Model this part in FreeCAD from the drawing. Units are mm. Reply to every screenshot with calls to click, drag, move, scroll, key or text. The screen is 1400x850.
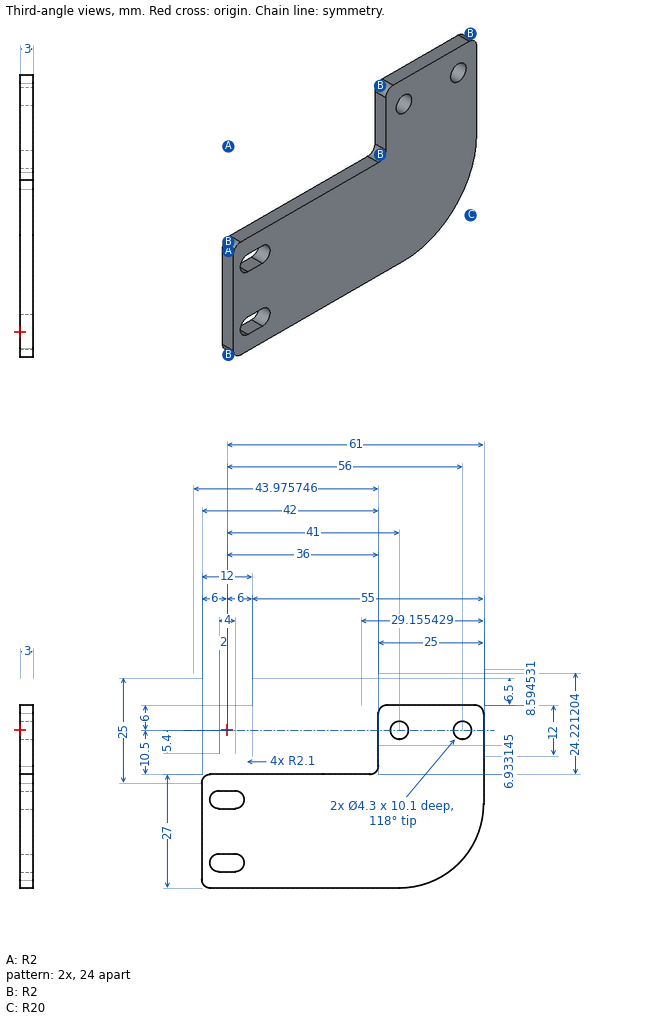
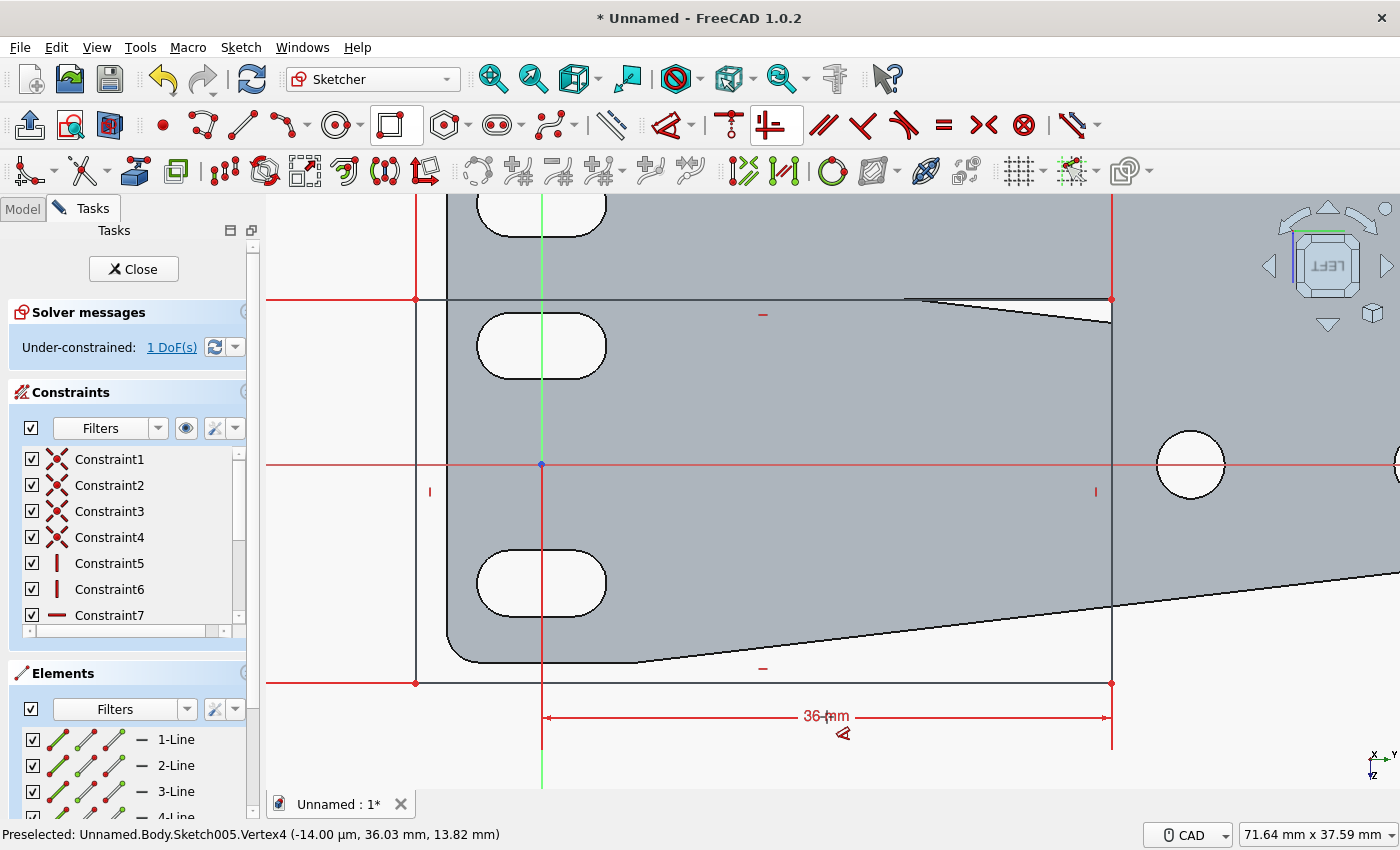
click(416, 300)
click(382, 382)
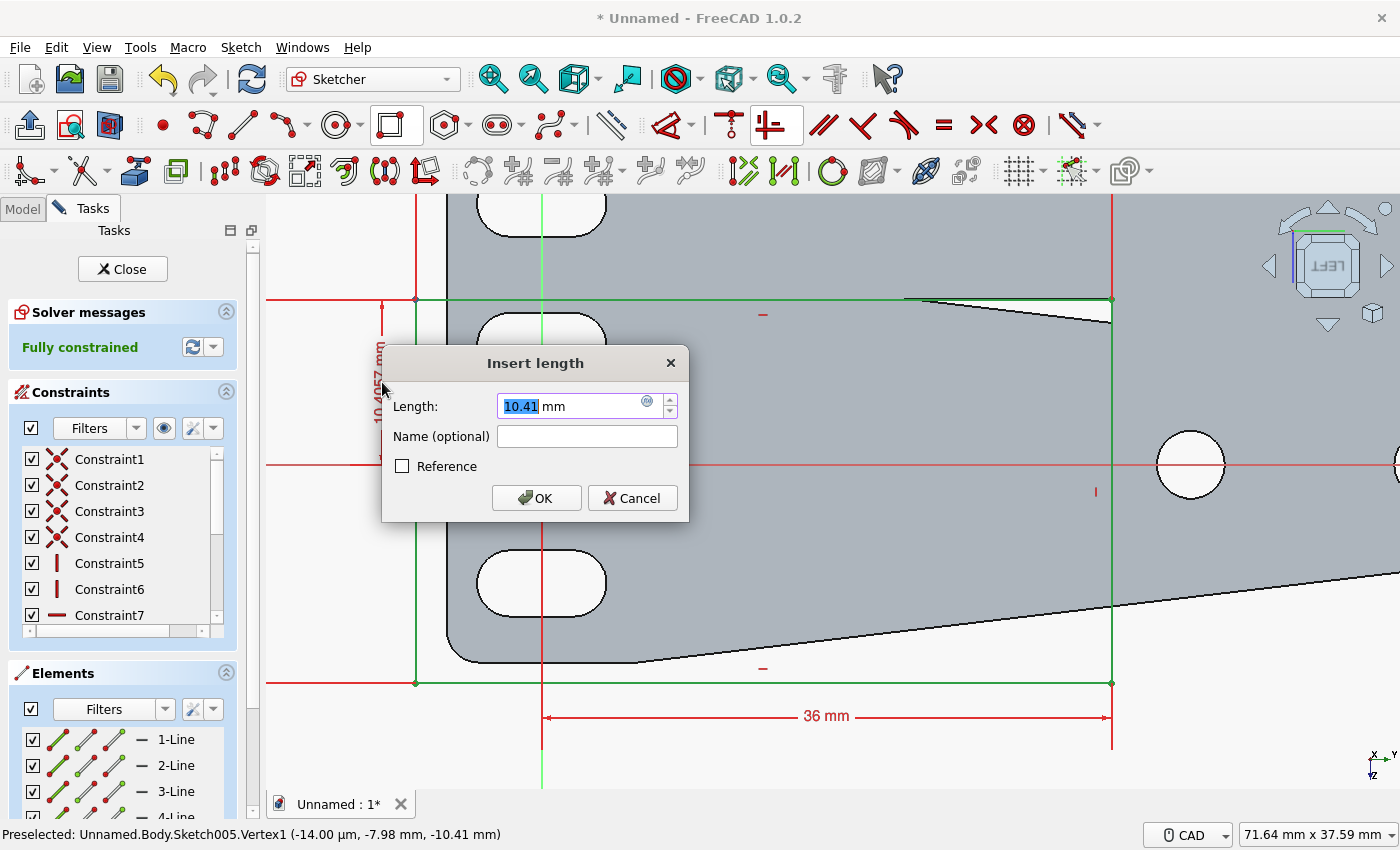
text(10.5)
key(Return)
key(Escape)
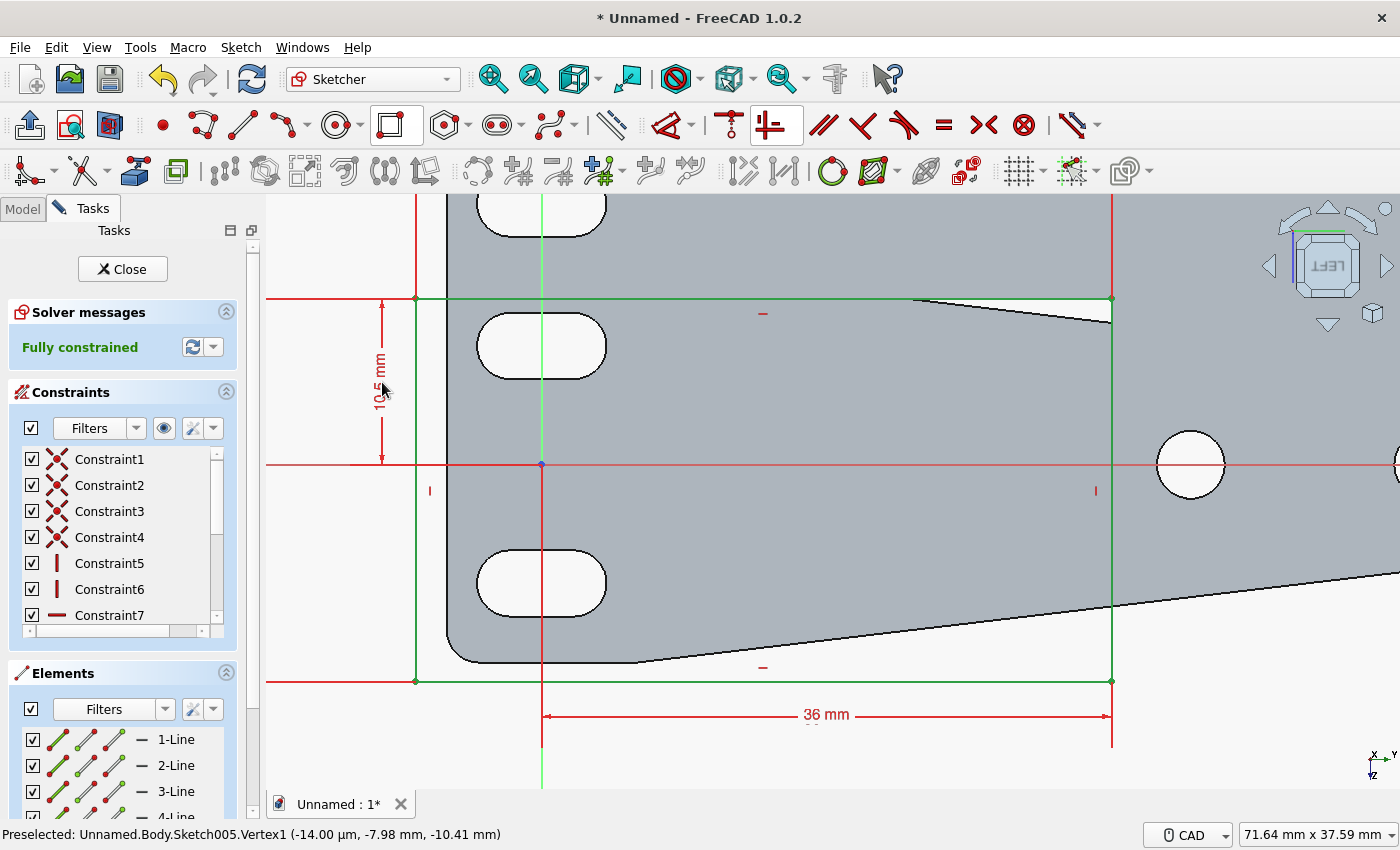
click(123, 269)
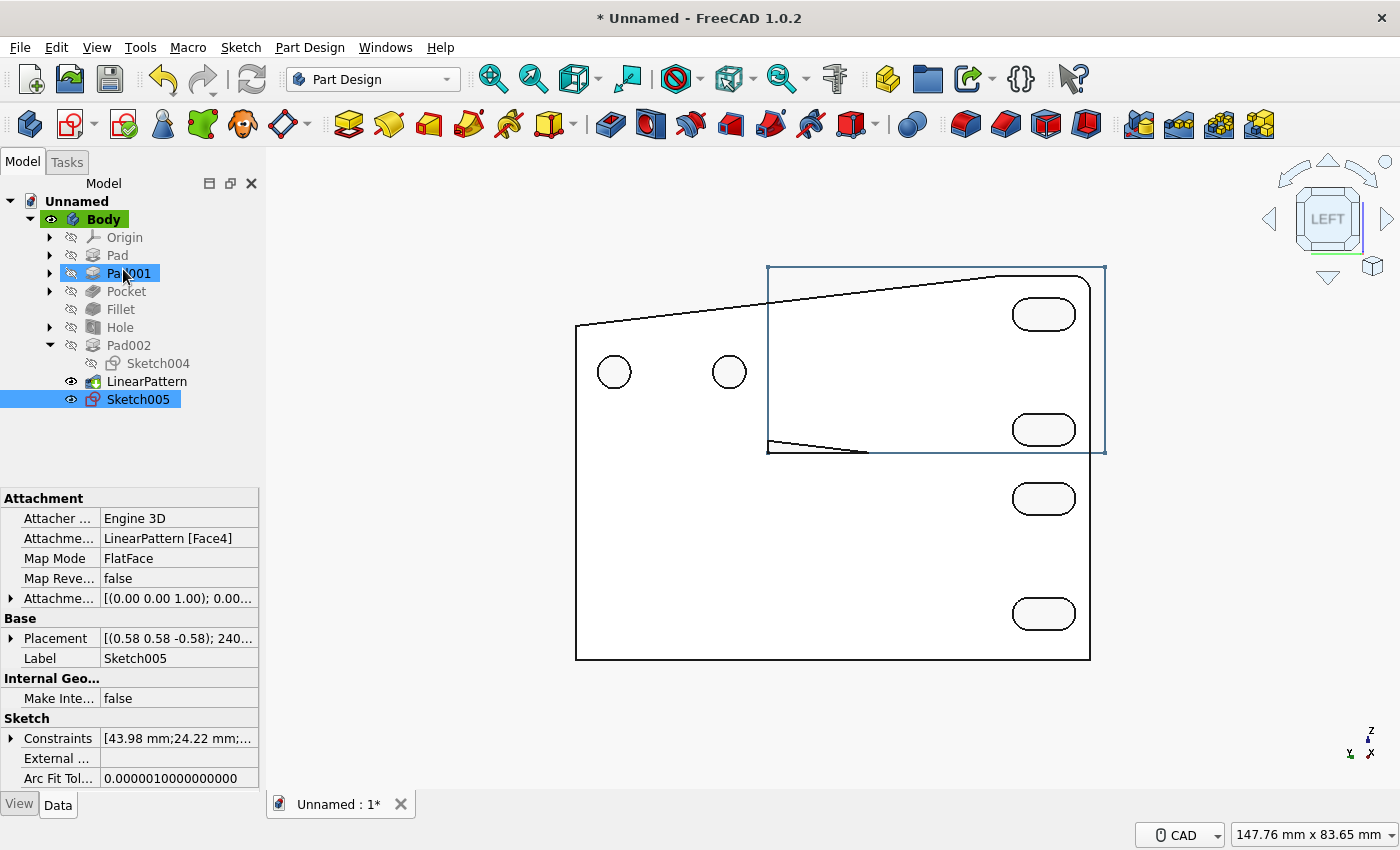
click(612, 124)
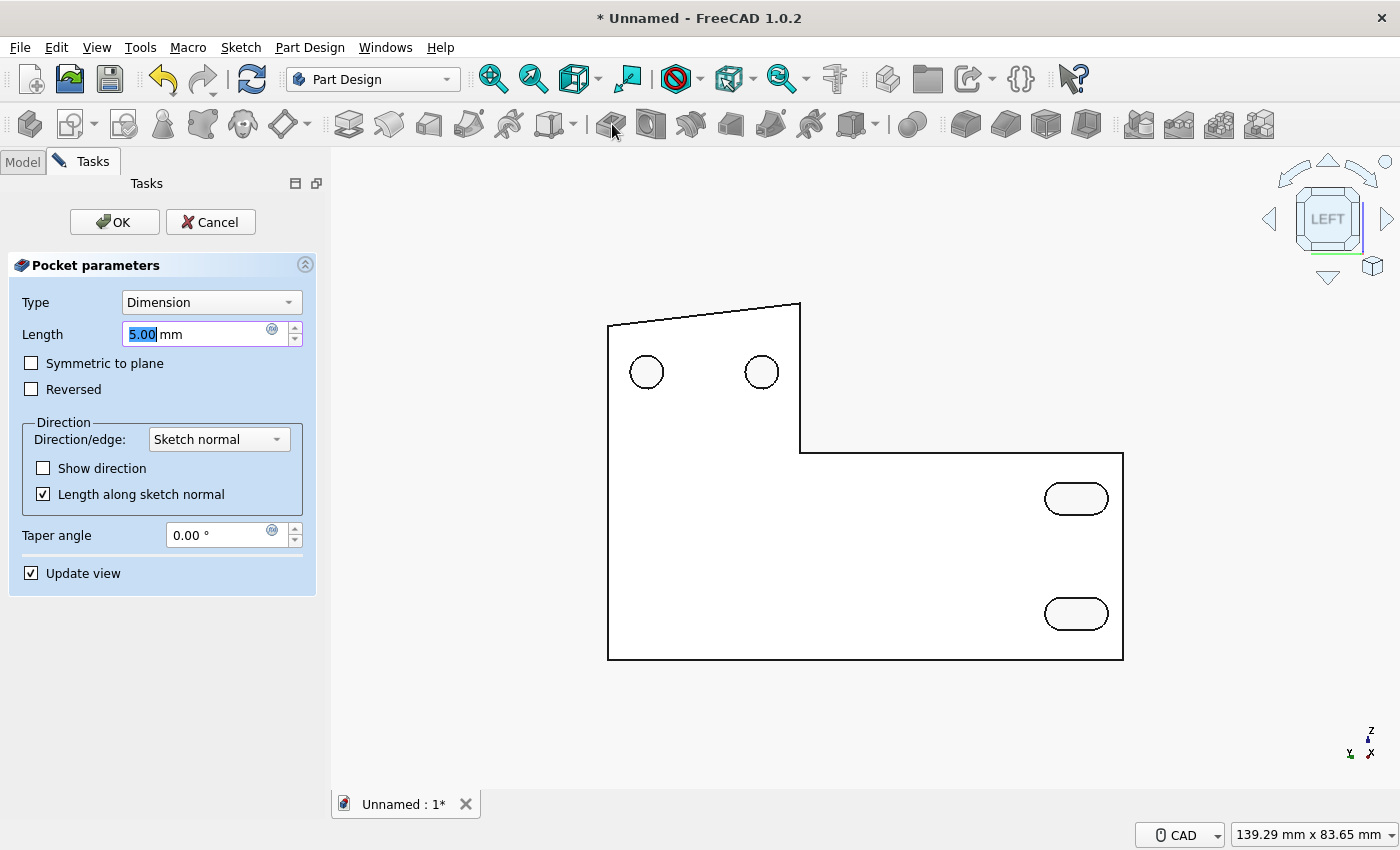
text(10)
key(Tab)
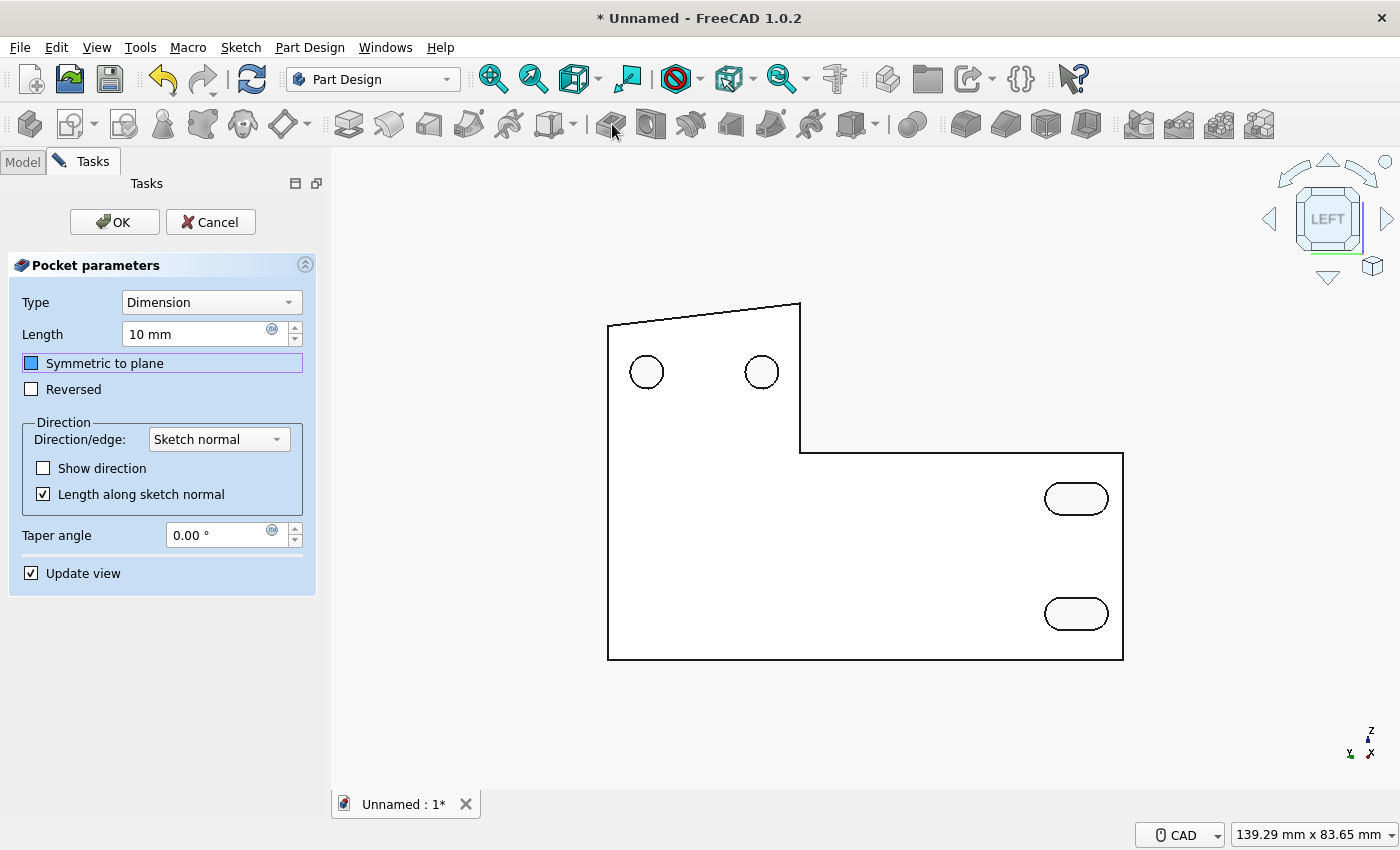
click(115, 222)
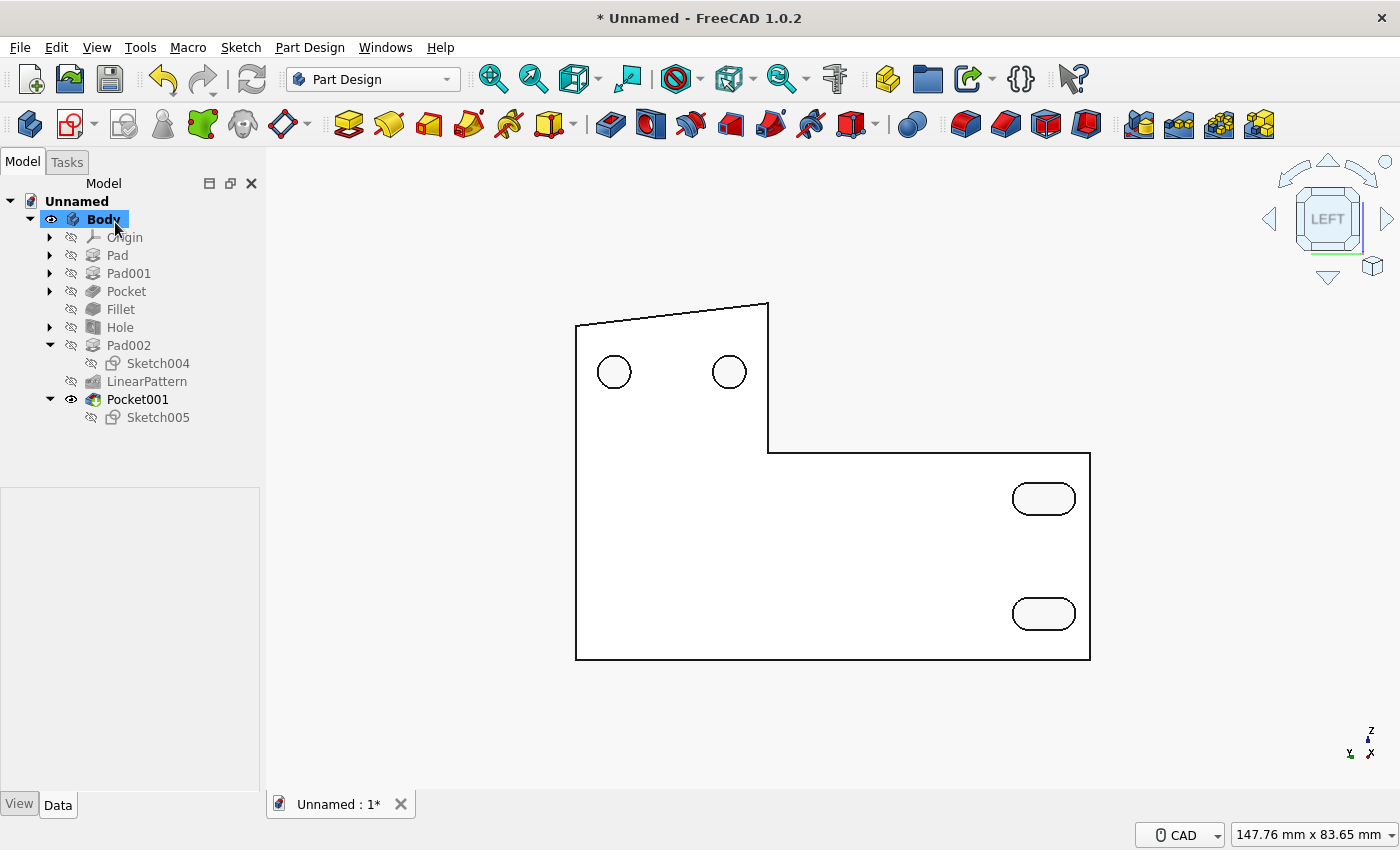
click(70, 124)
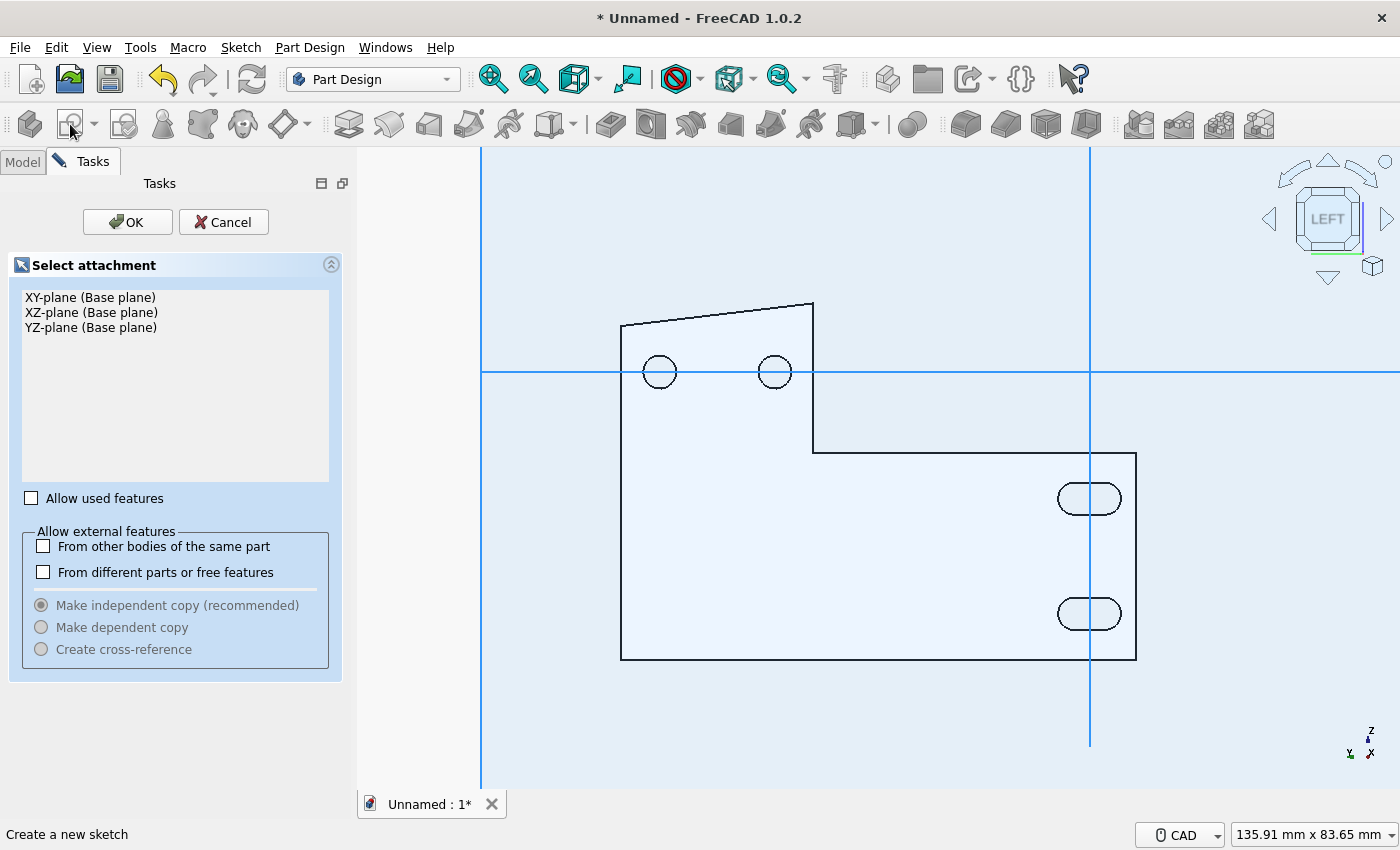
click(82, 328)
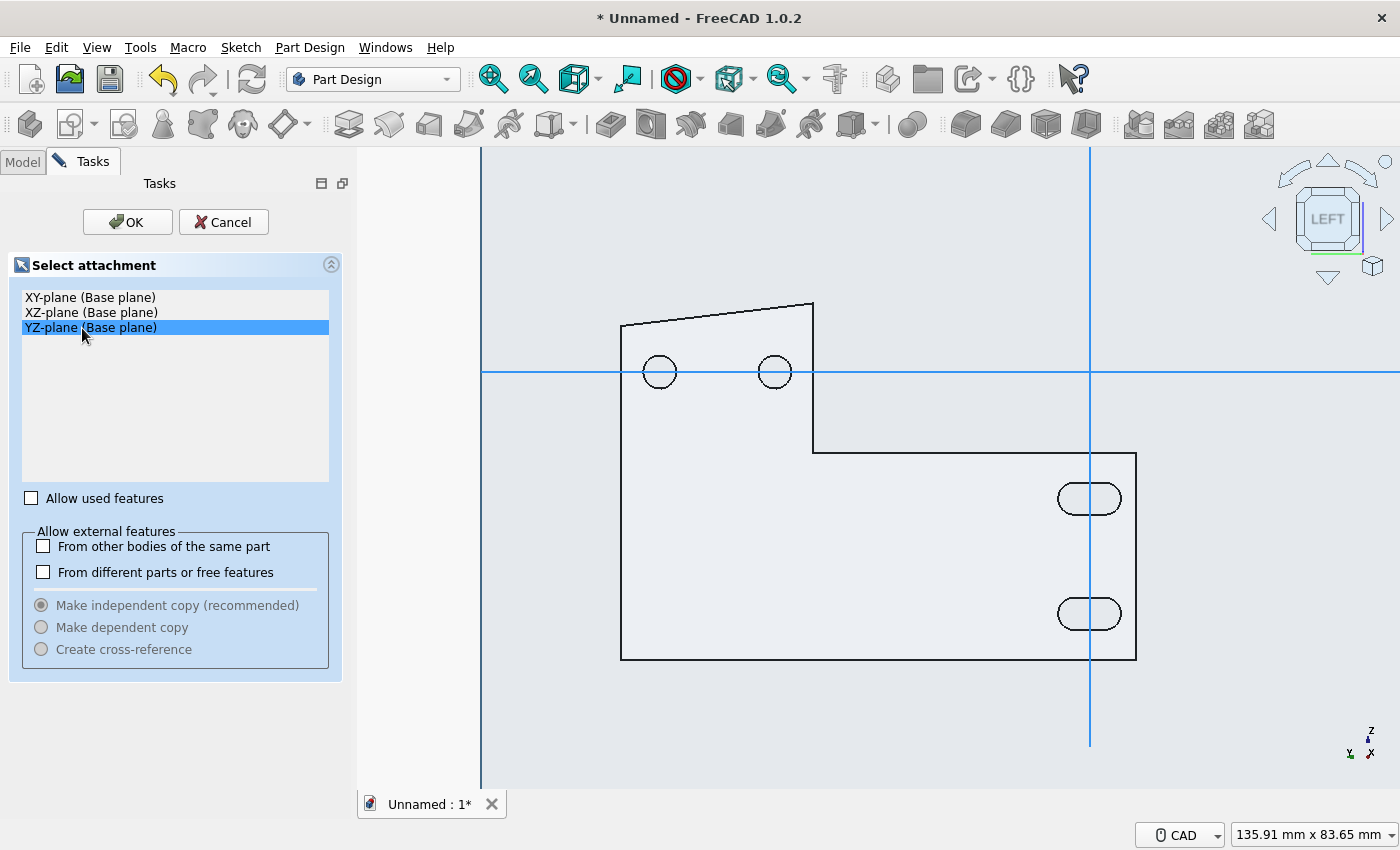
click(128, 222)